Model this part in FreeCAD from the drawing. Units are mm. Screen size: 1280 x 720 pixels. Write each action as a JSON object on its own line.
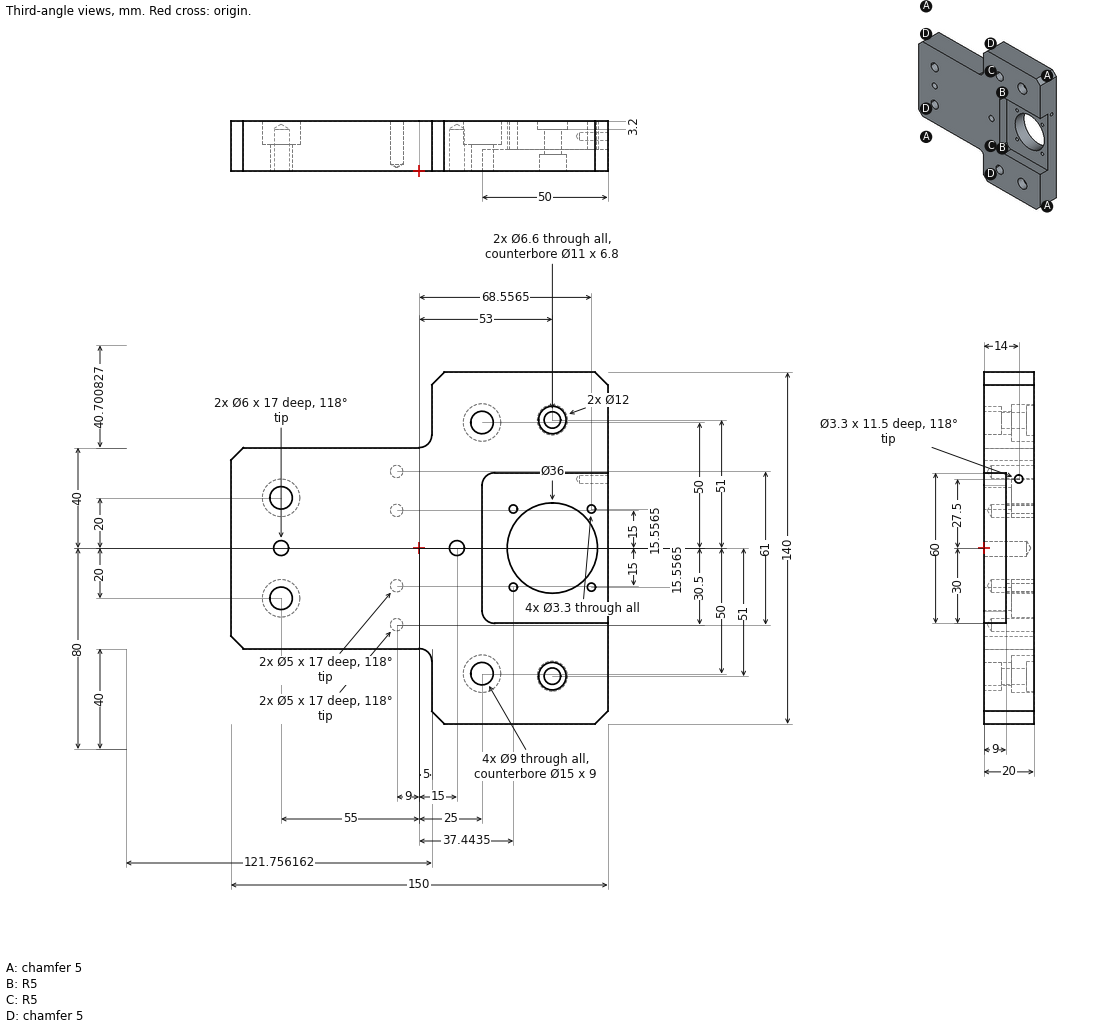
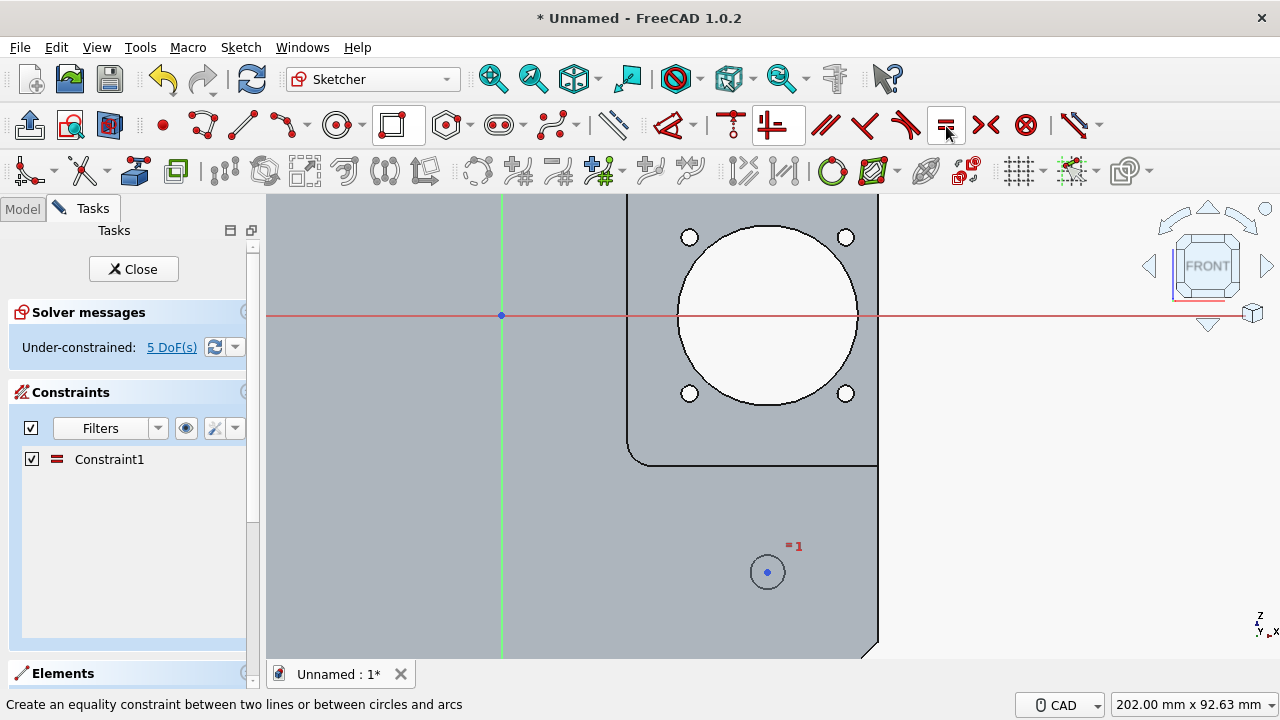
{"action": "scroll", "coordinate": [779, 561], "scroll_direction": "down", "scroll_amount": 3}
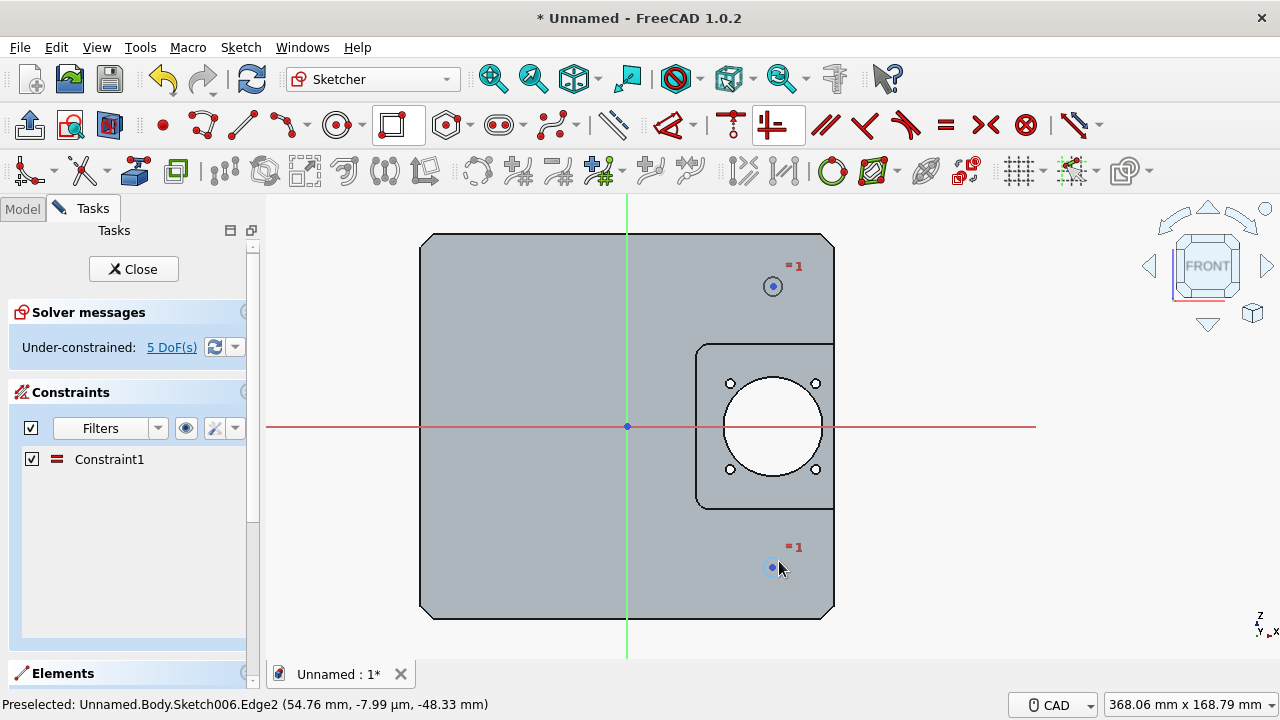
{"action": "left_click", "coordinate": [773, 287]}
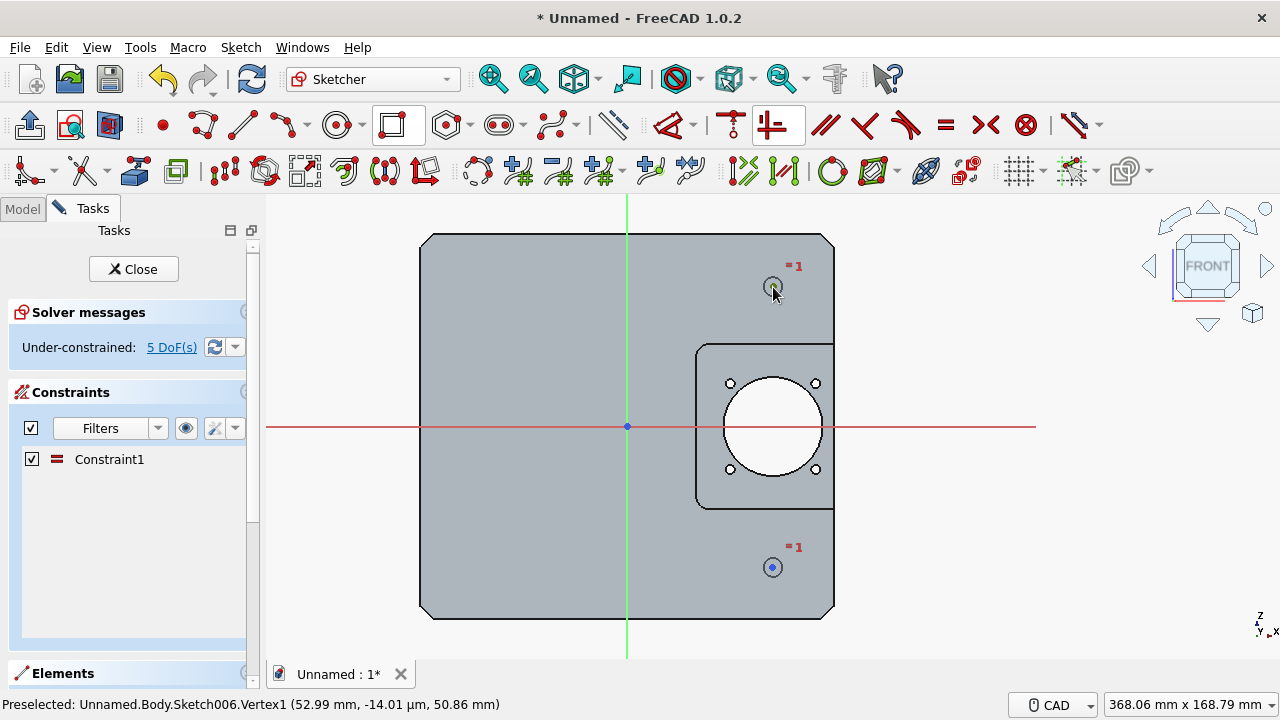
{"action": "left_click", "coordinate": [773, 567]}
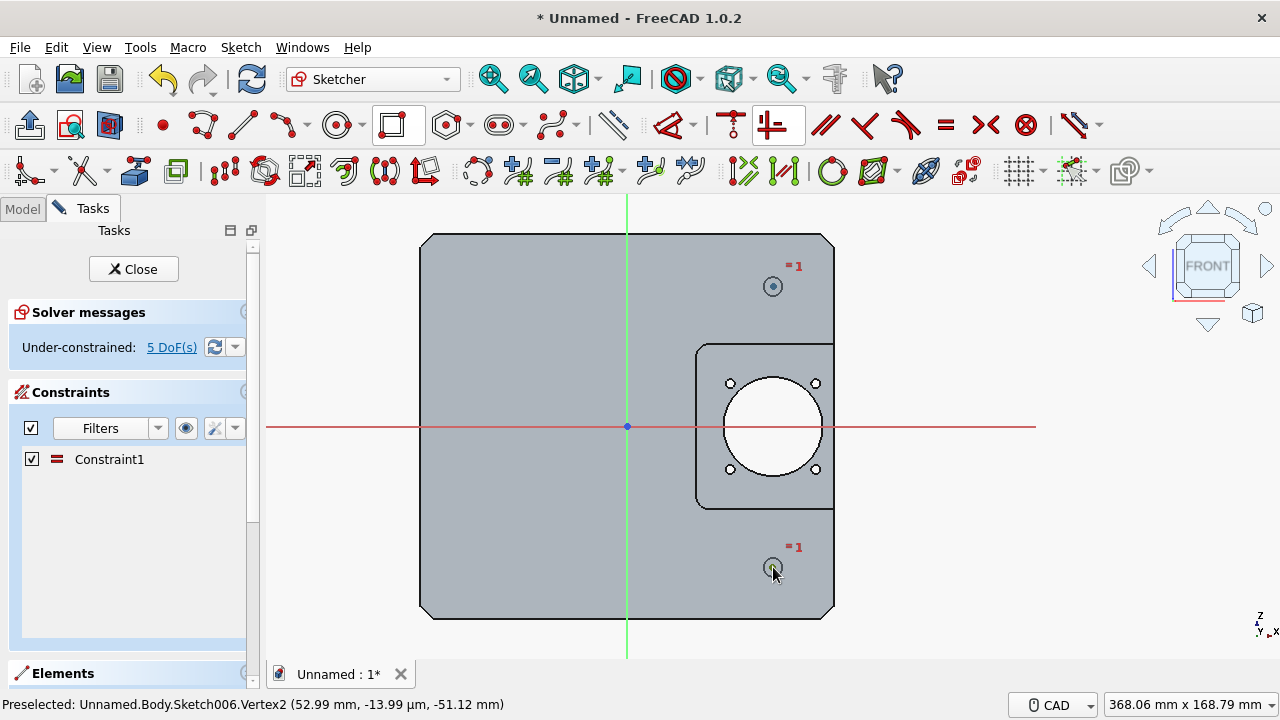
{"action": "key", "text": "v"}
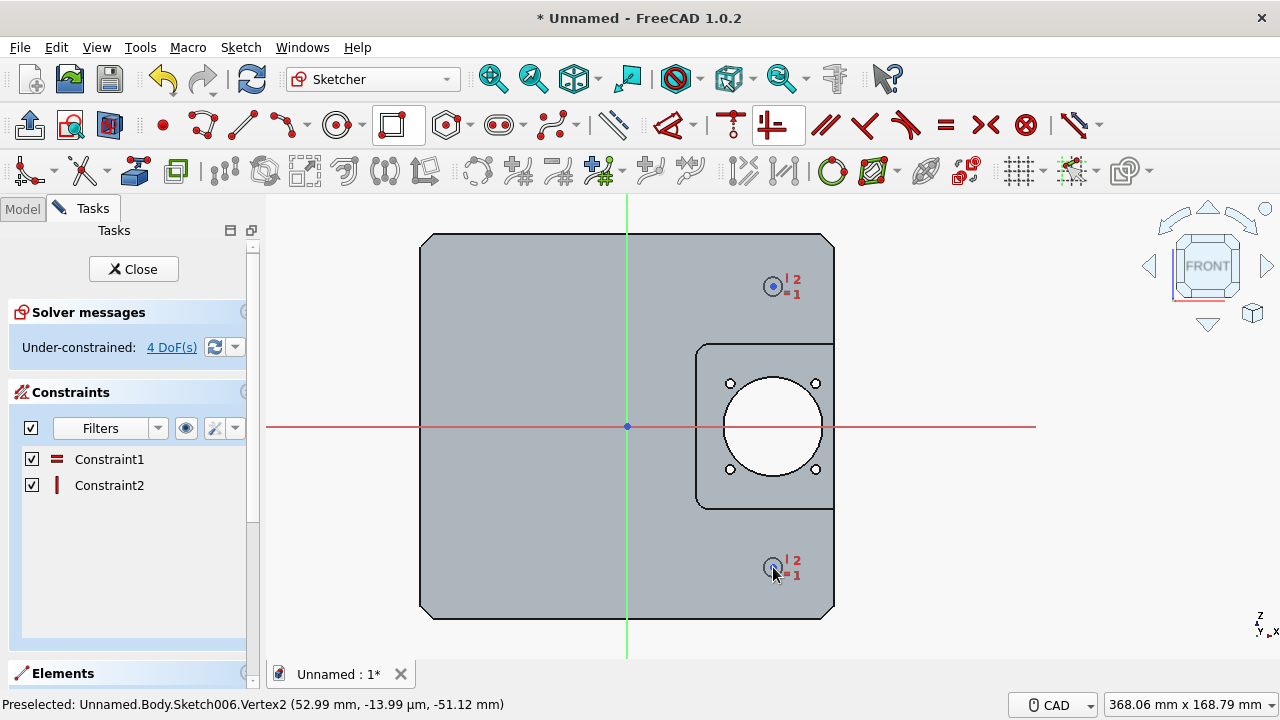
{"action": "left_click", "coordinate": [668, 126]}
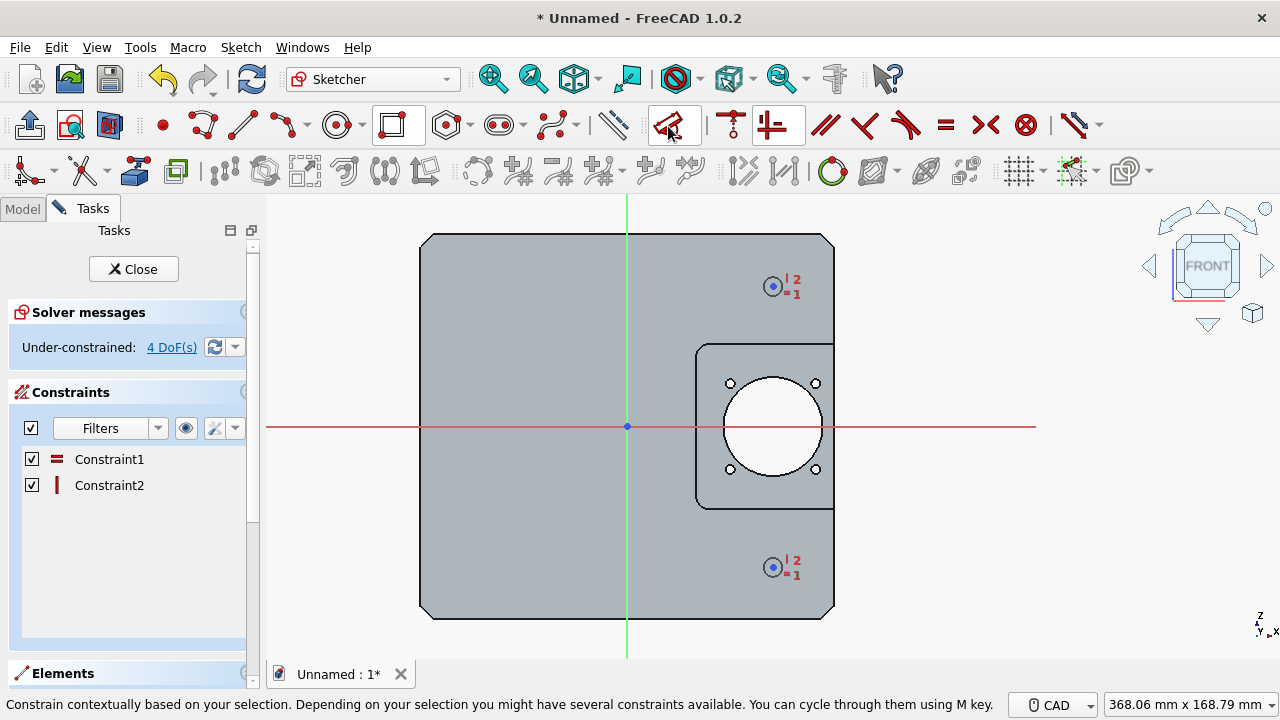
{"action": "scroll", "coordinate": [780, 280], "scroll_direction": "up", "scroll_amount": 4}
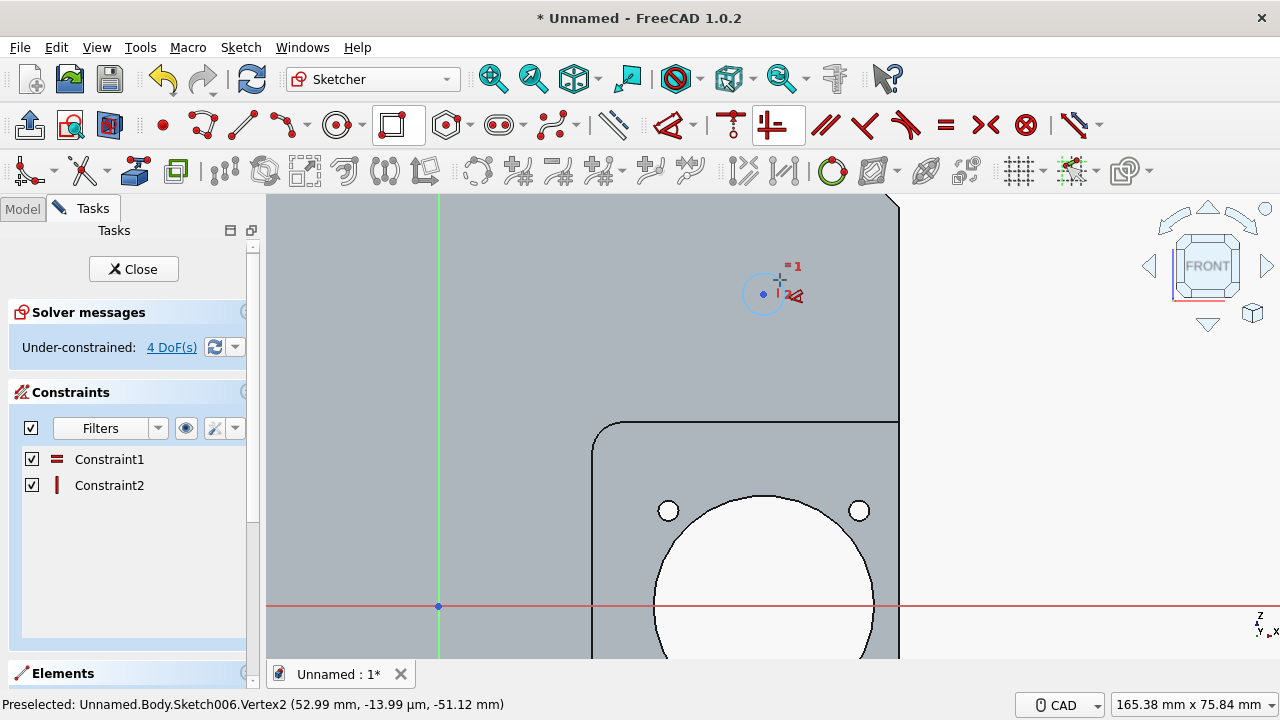
{"action": "left_click", "coordinate": [778, 280]}
{"action": "left_click", "coordinate": [801, 257]}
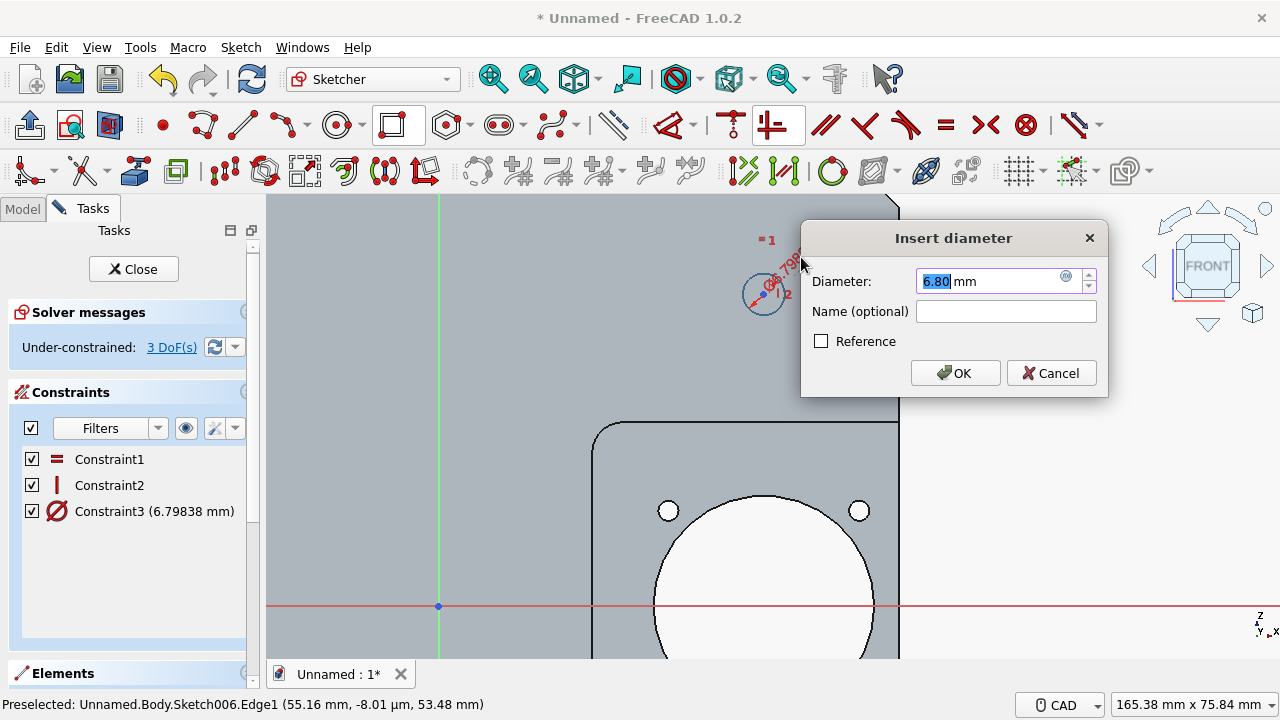
{"action": "type", "text": "6.6"}
{"action": "key", "text": "Return"}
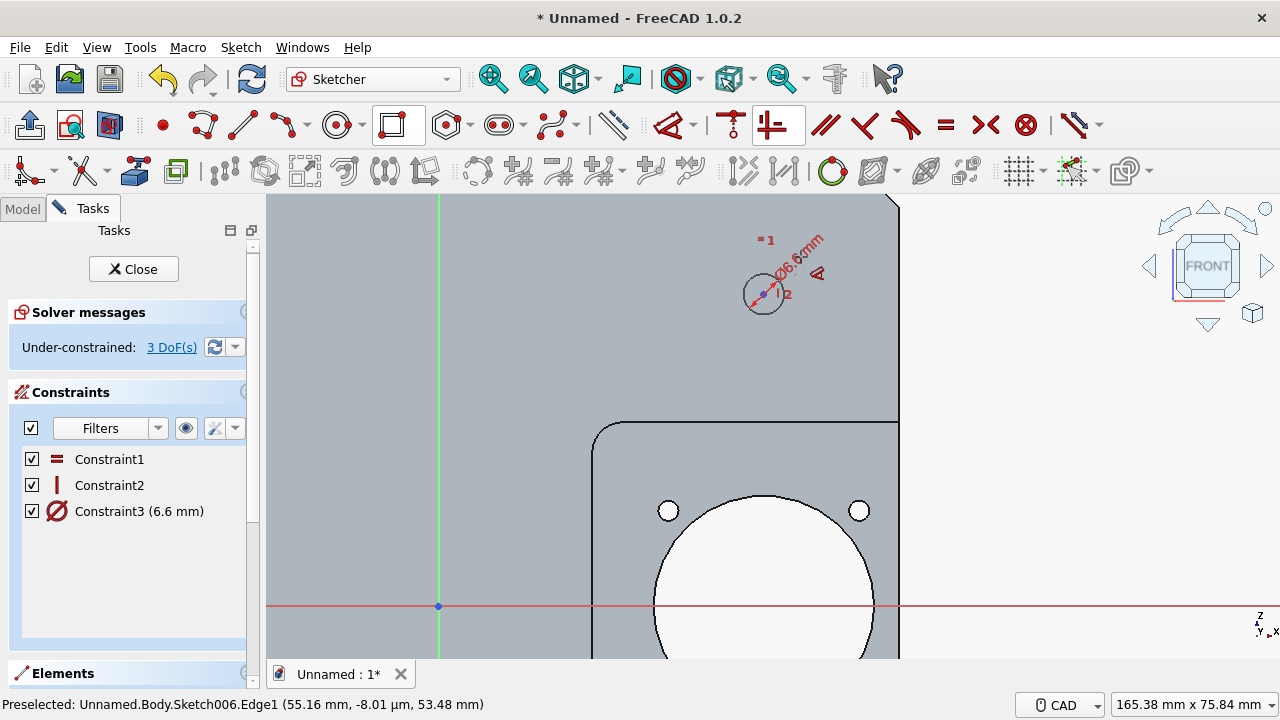
{"action": "left_click", "coordinate": [764, 294]}
{"action": "left_click", "coordinate": [601, 260]}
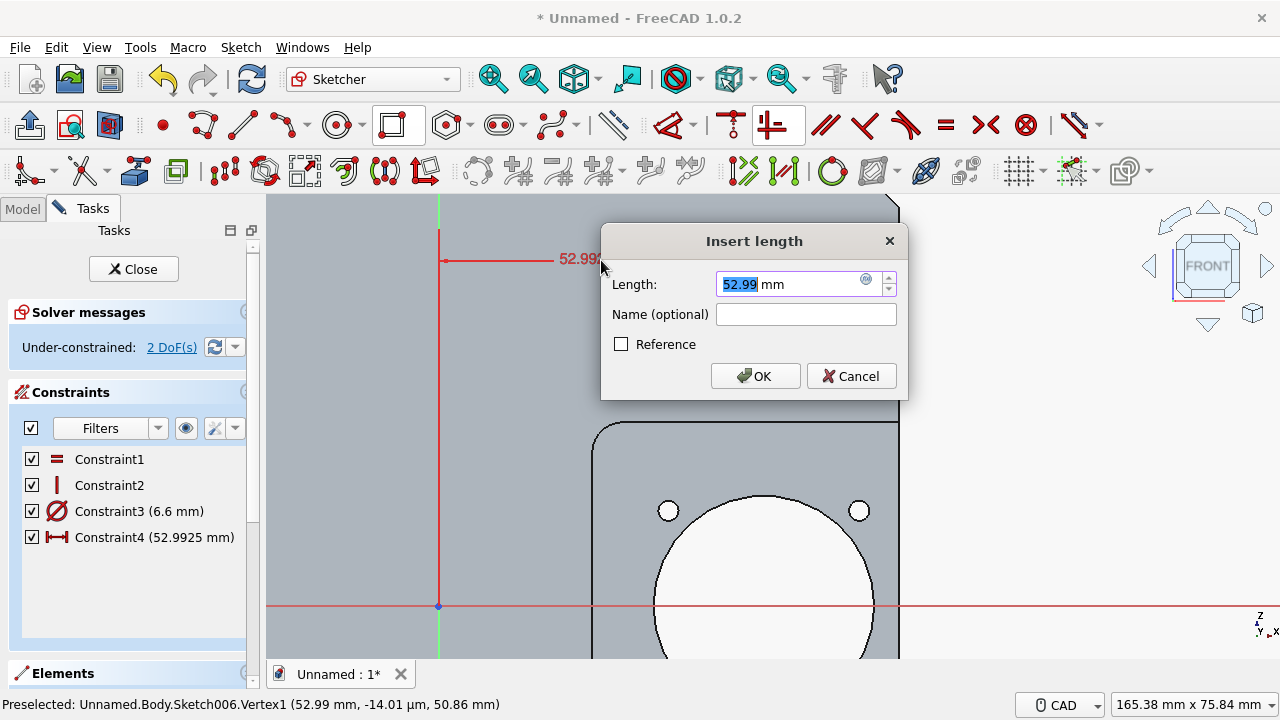
{"action": "type", "text": "53"}
{"action": "key", "text": "Return"}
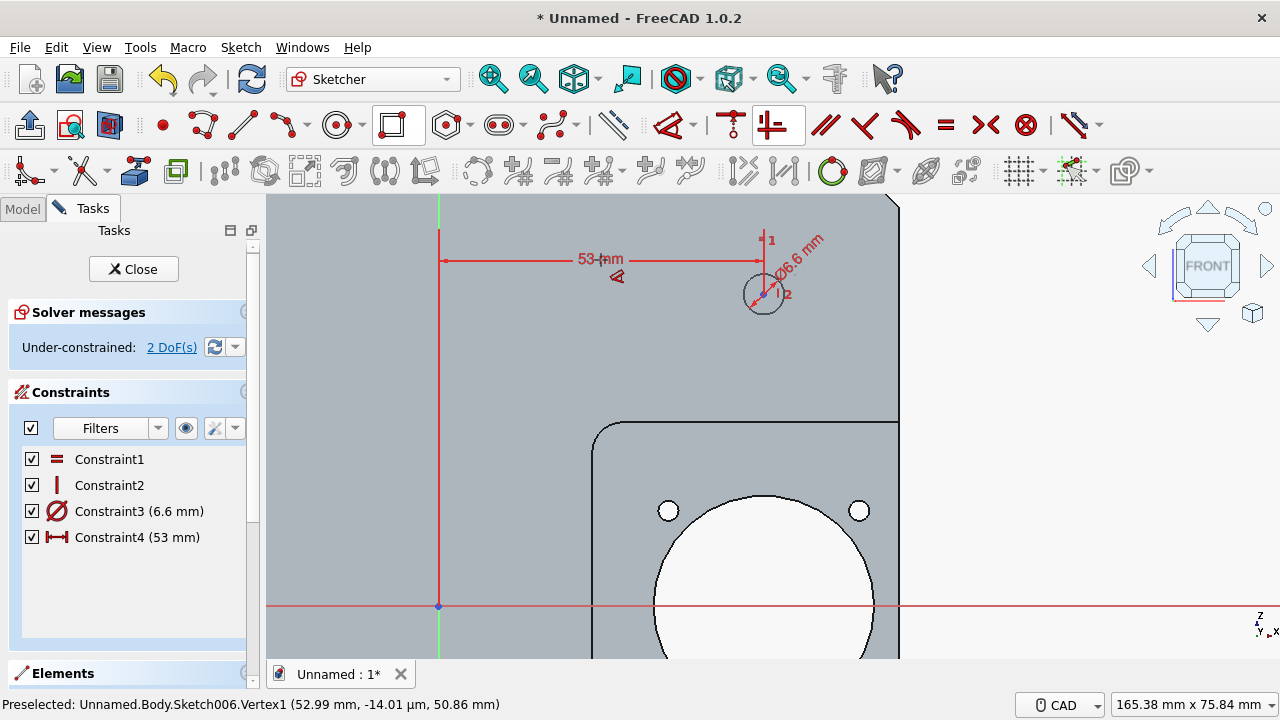
{"action": "left_click", "coordinate": [764, 294]}
{"action": "left_click", "coordinate": [405, 450]}